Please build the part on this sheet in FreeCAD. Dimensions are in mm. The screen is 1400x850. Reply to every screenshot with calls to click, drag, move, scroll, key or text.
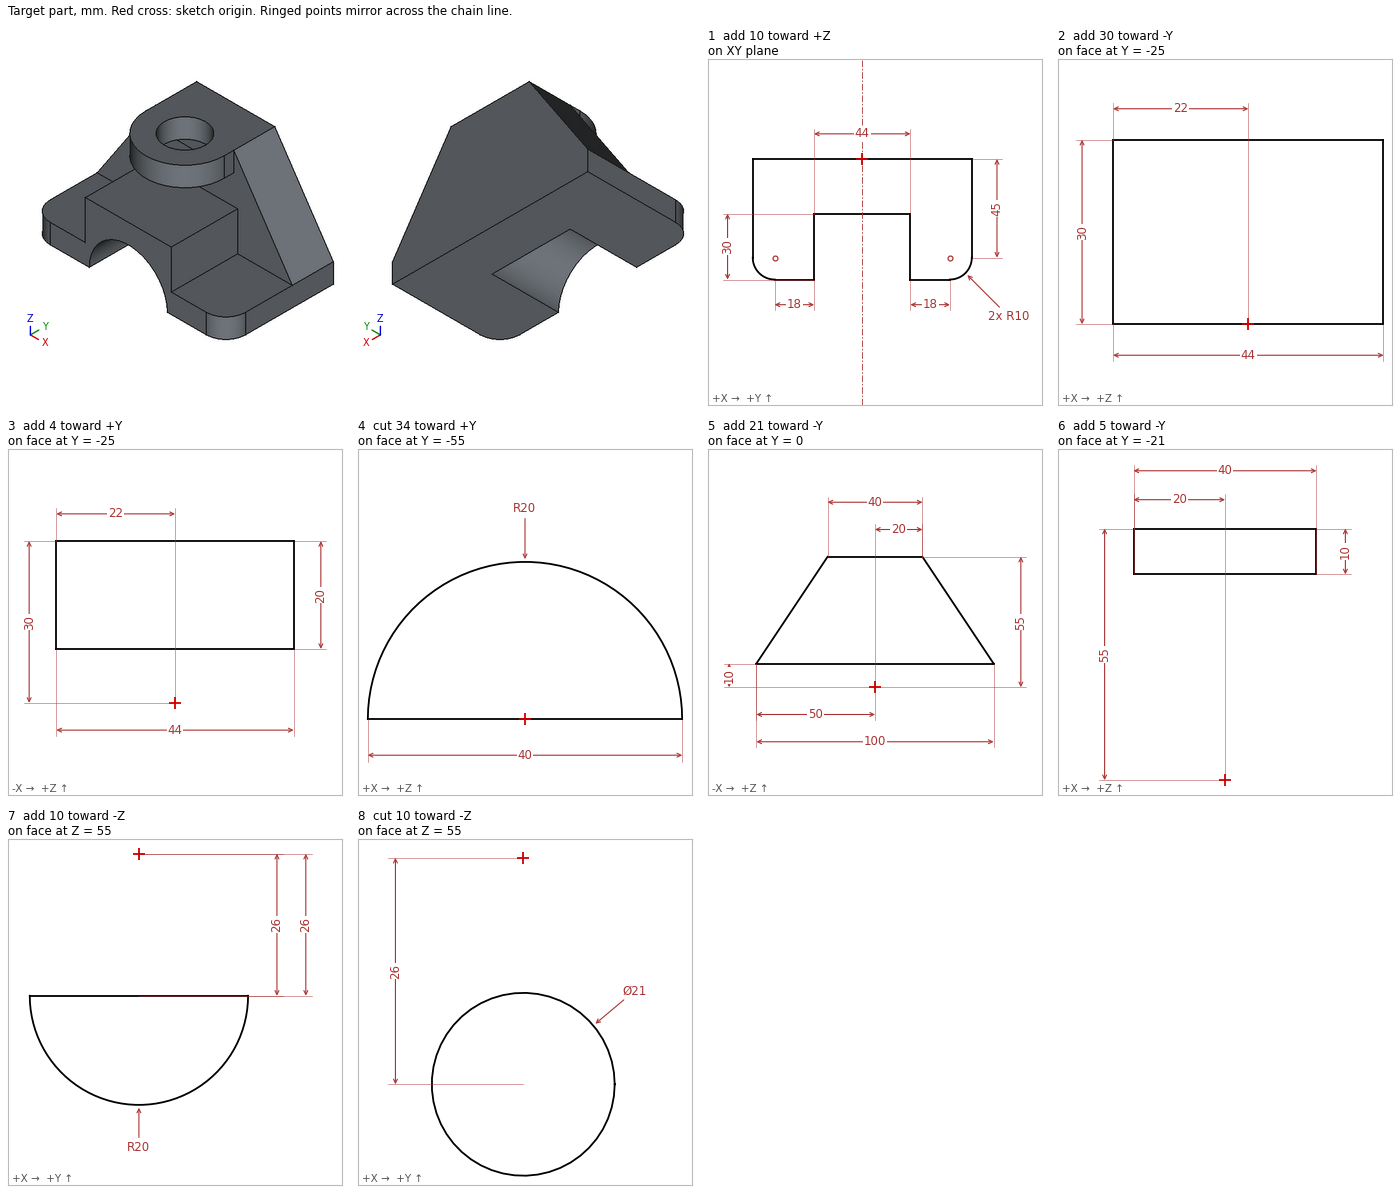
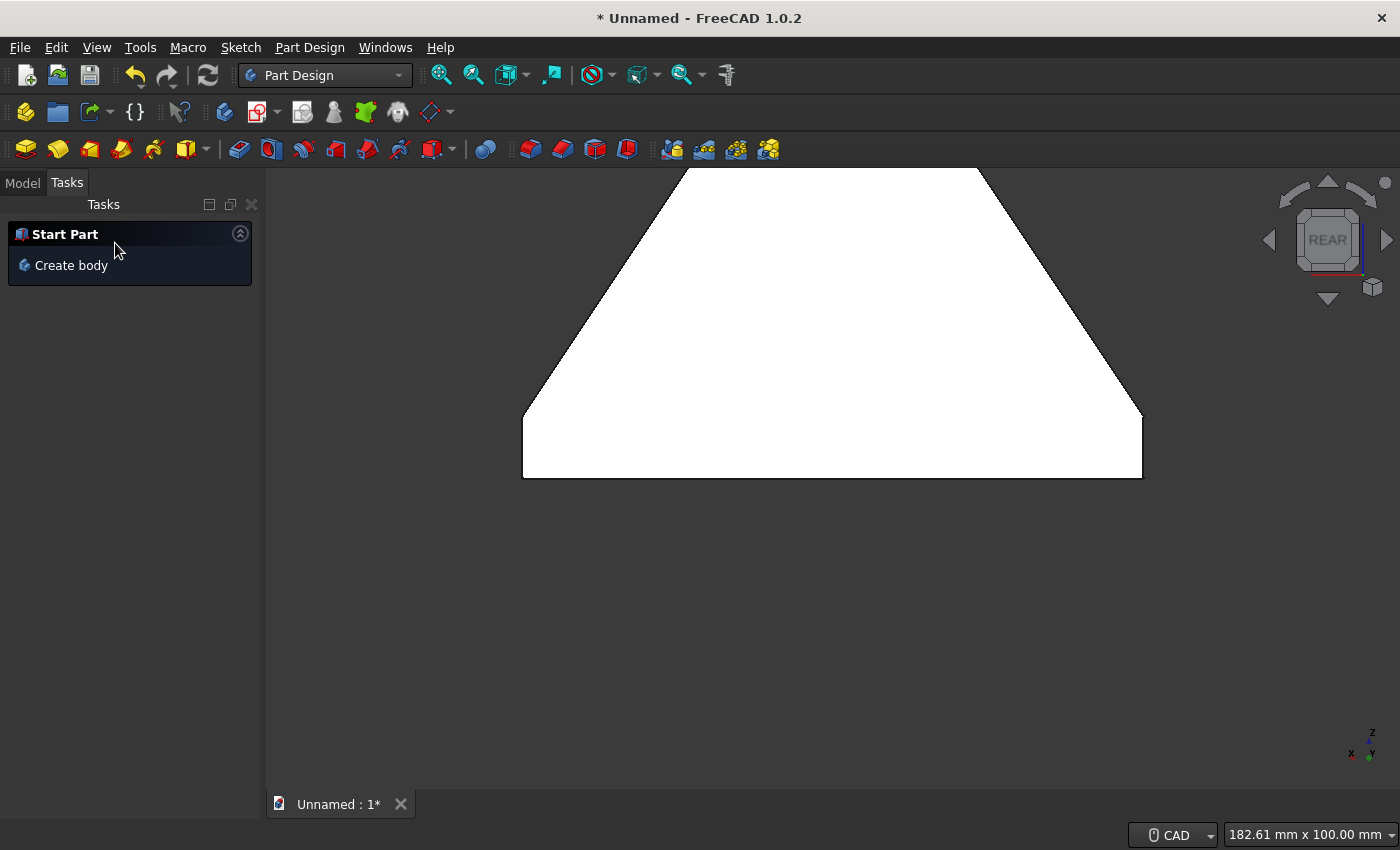
click(442, 76)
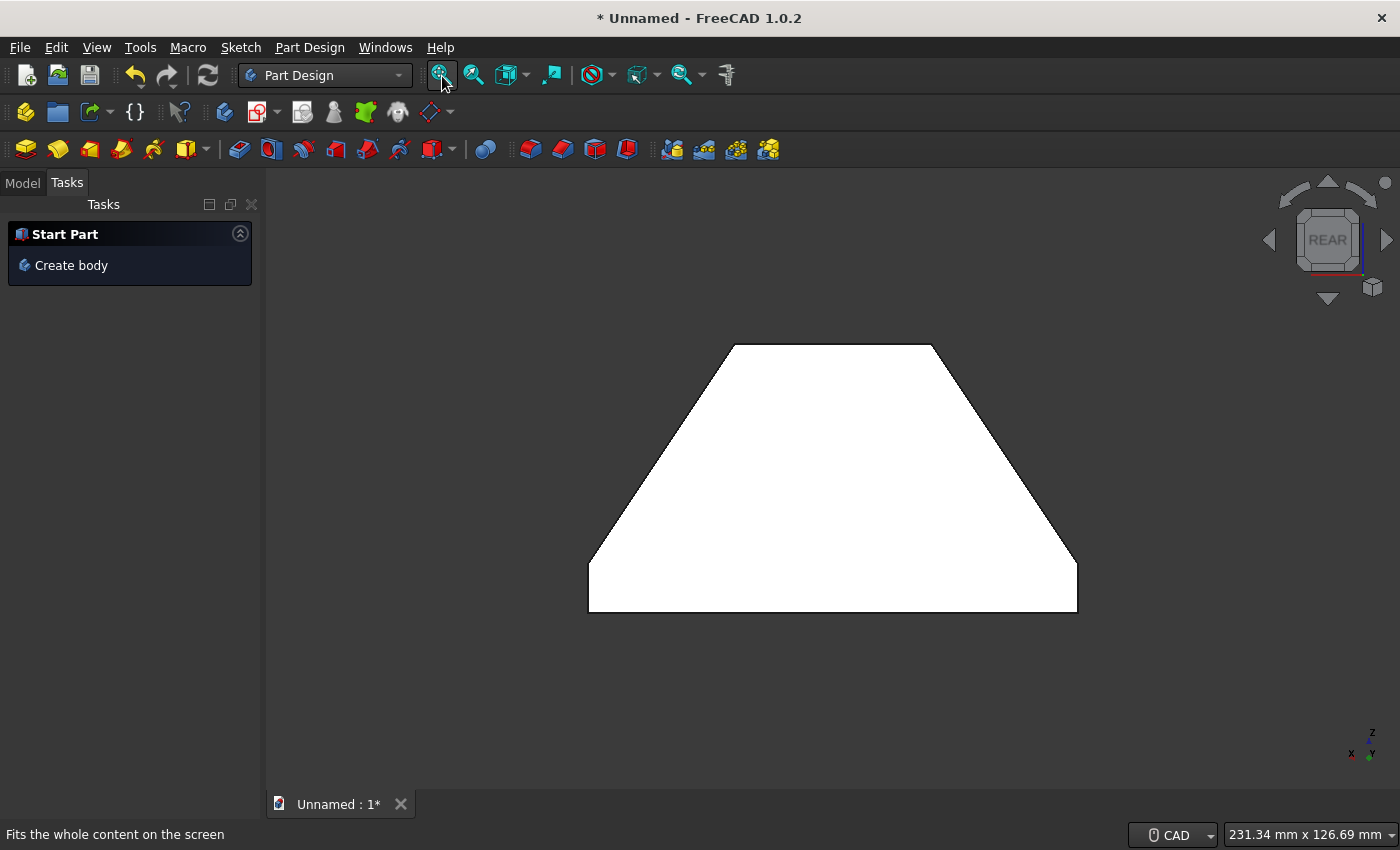
key(0)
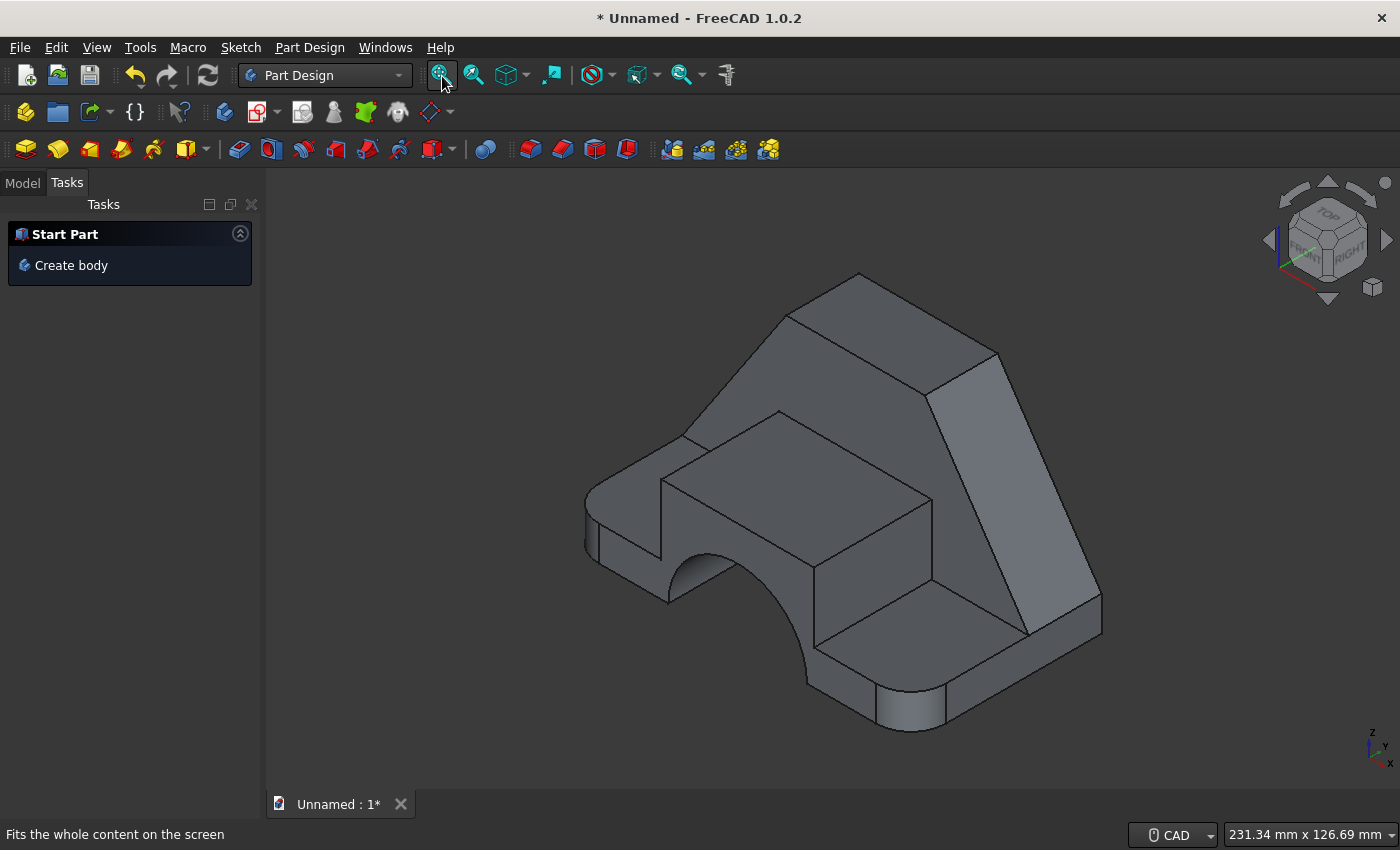
click(905, 422)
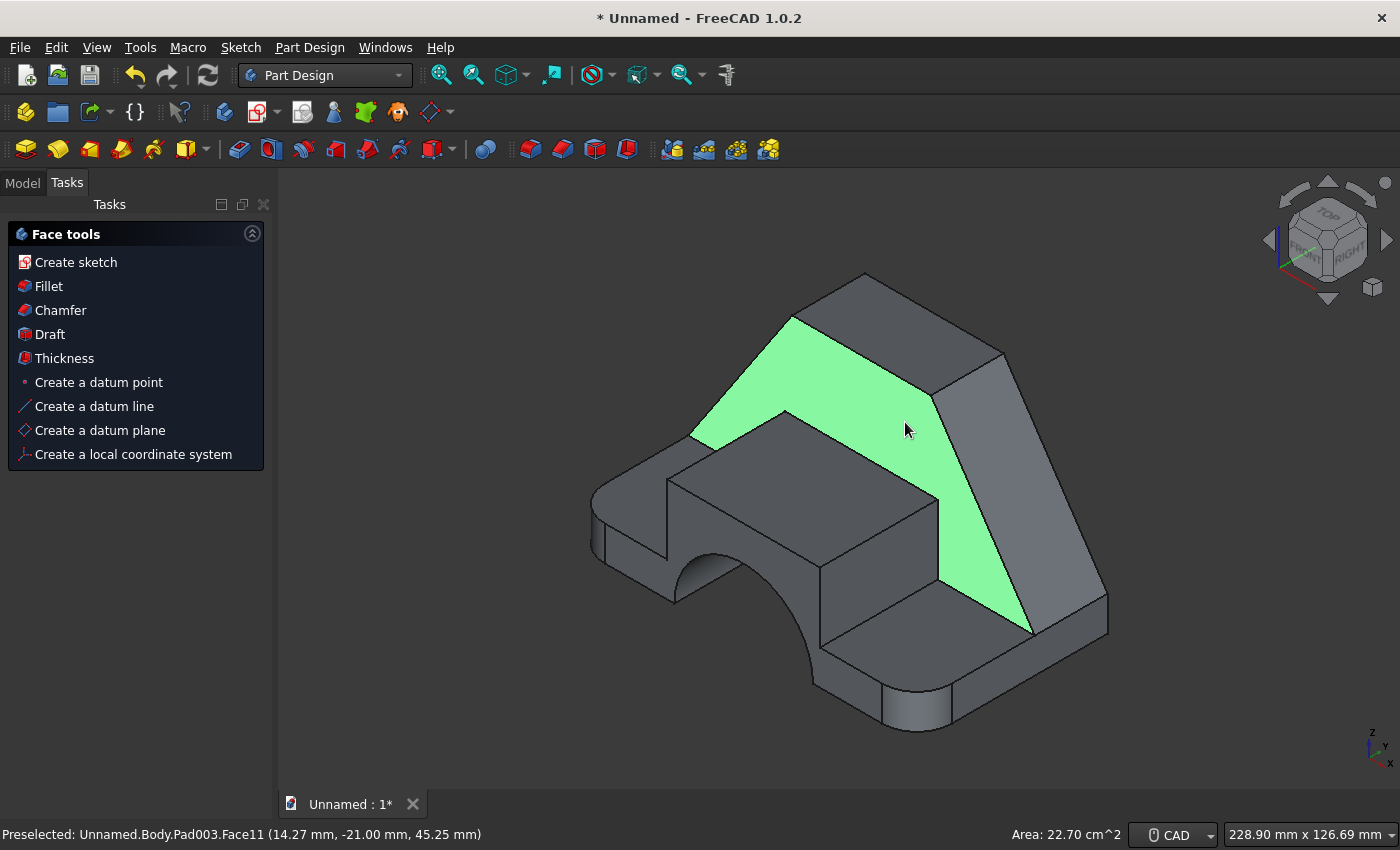
click(258, 112)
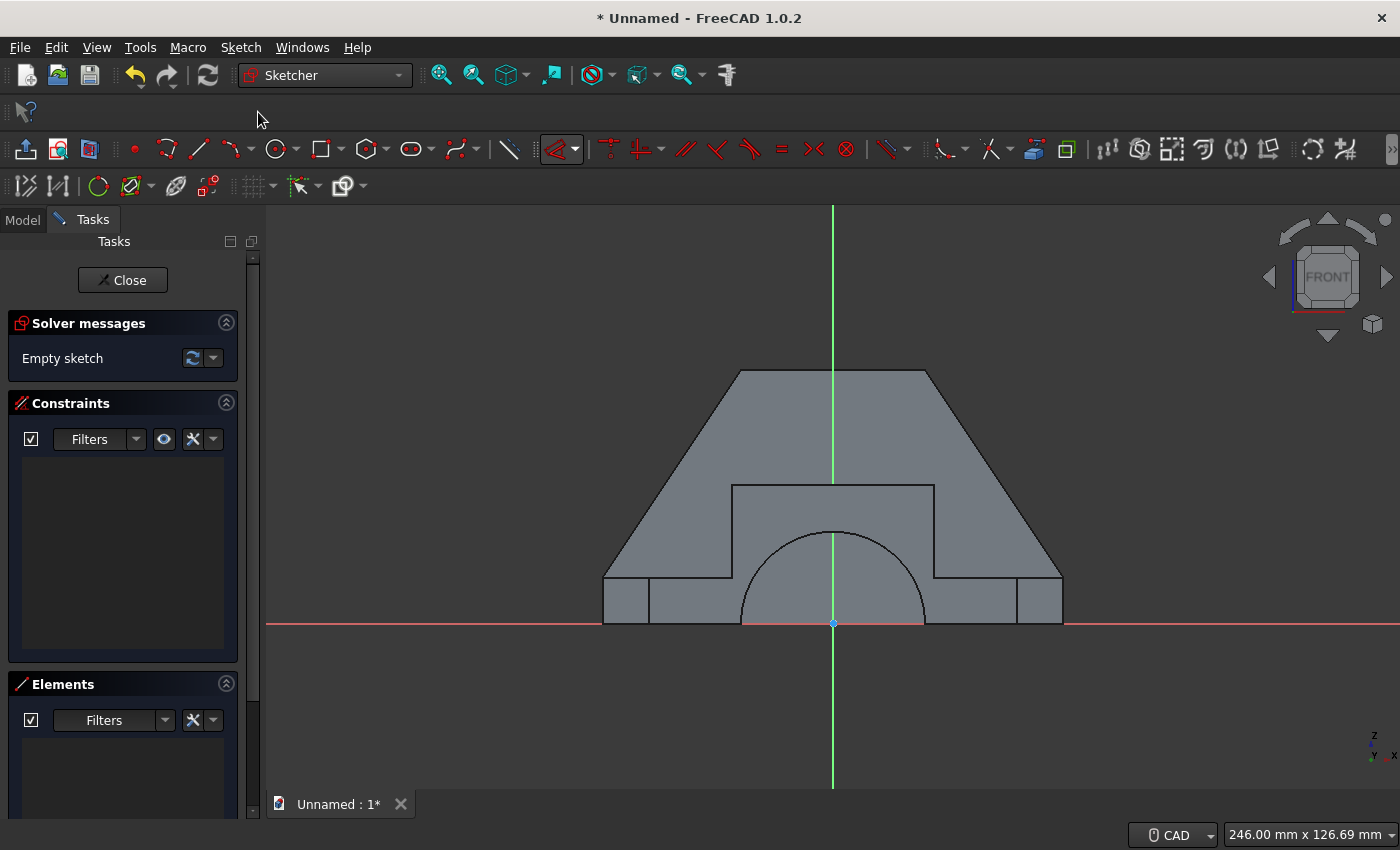
scroll(972, 497, up, 2)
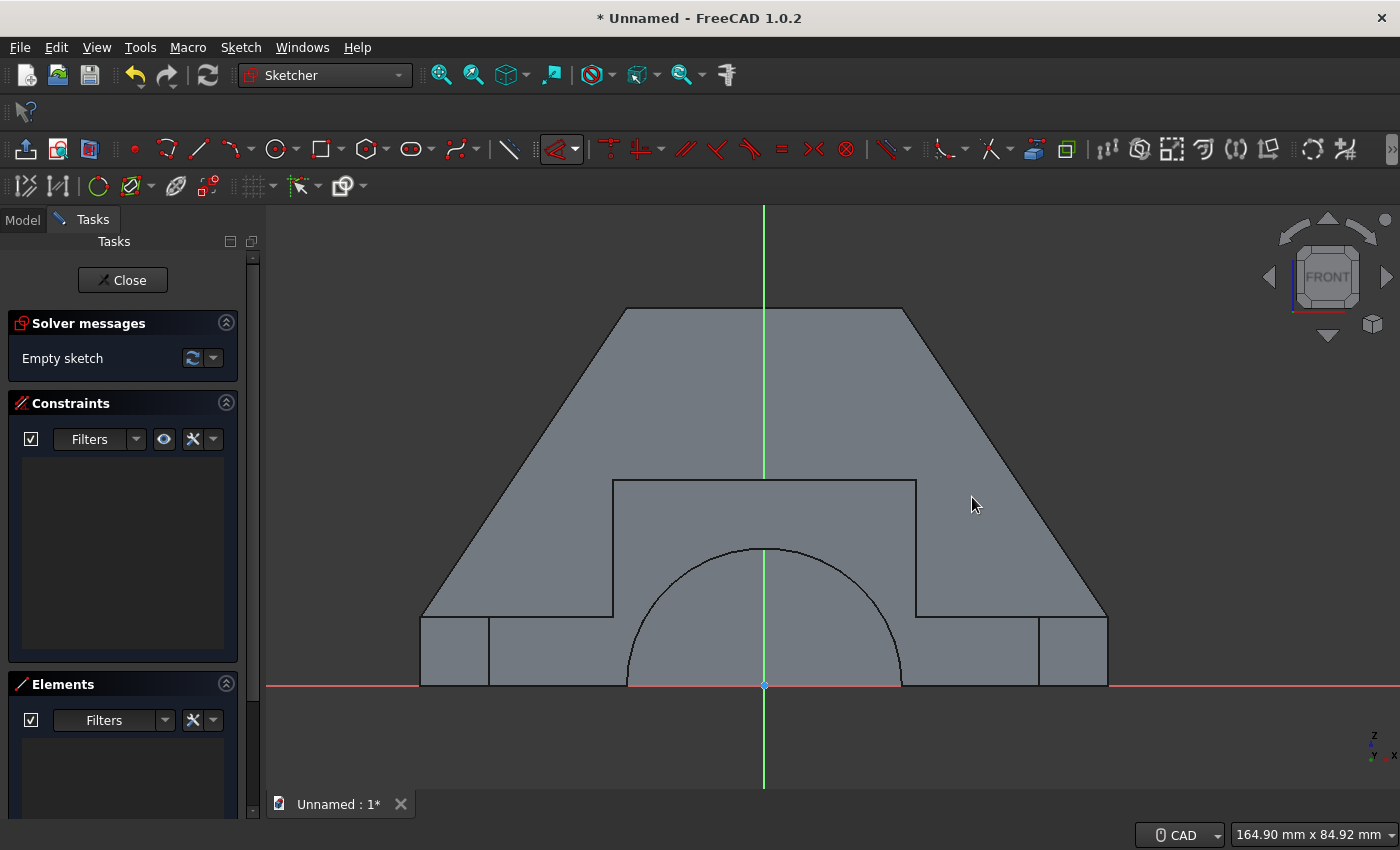
click(322, 150)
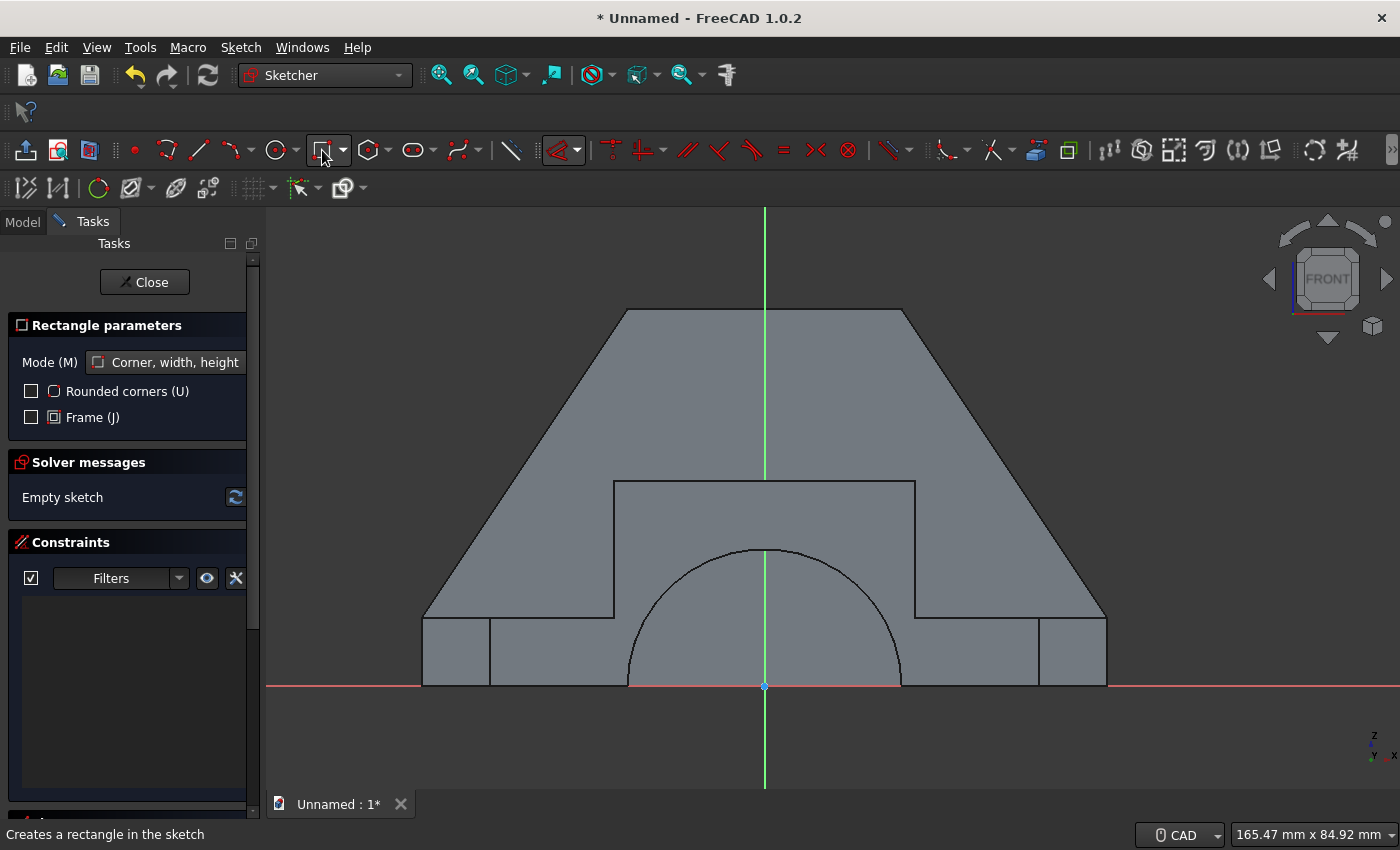
click(627, 309)
move(902, 378)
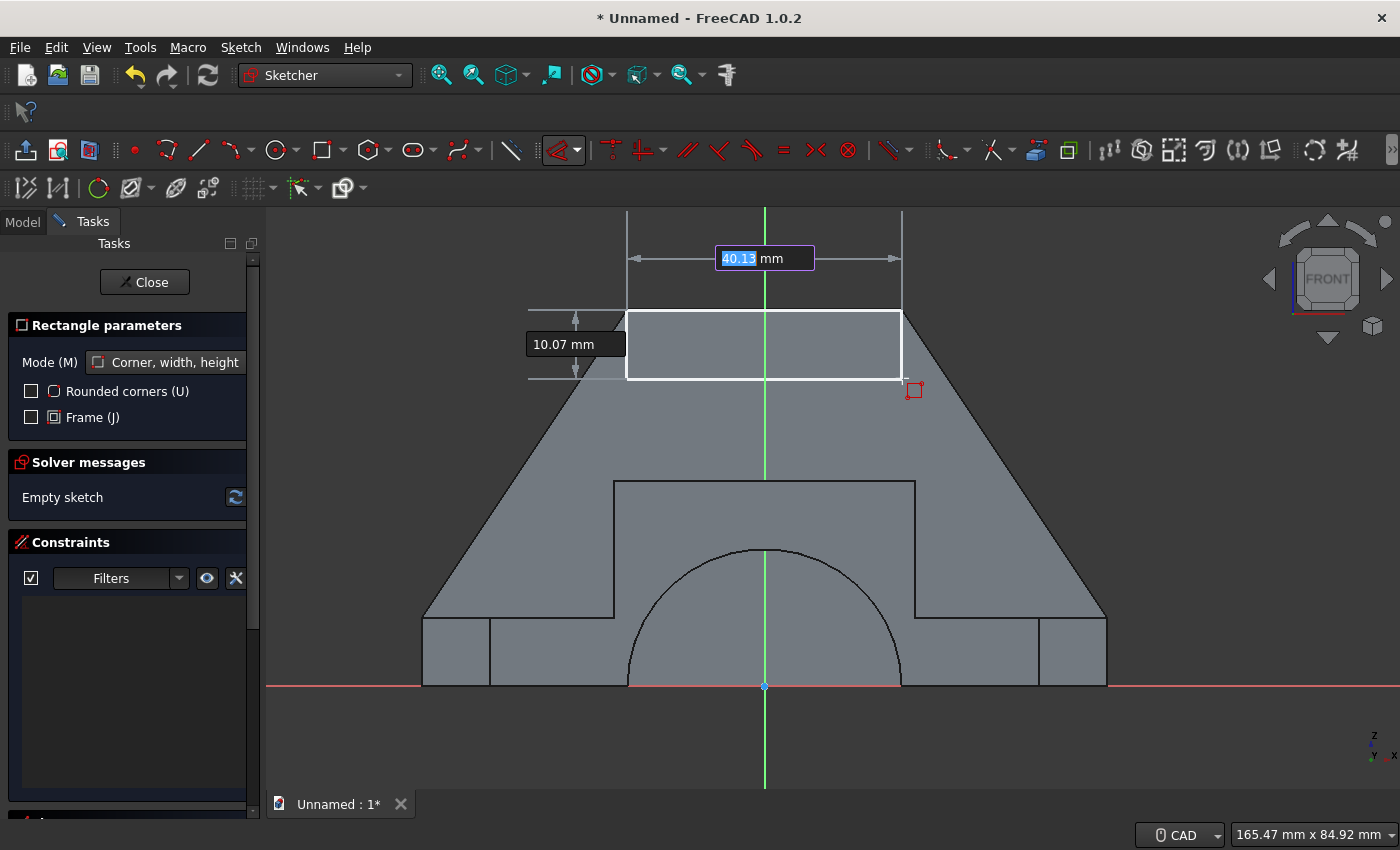
text(40)
key(Tab)
text(10)
key(Return)
key(Escape)